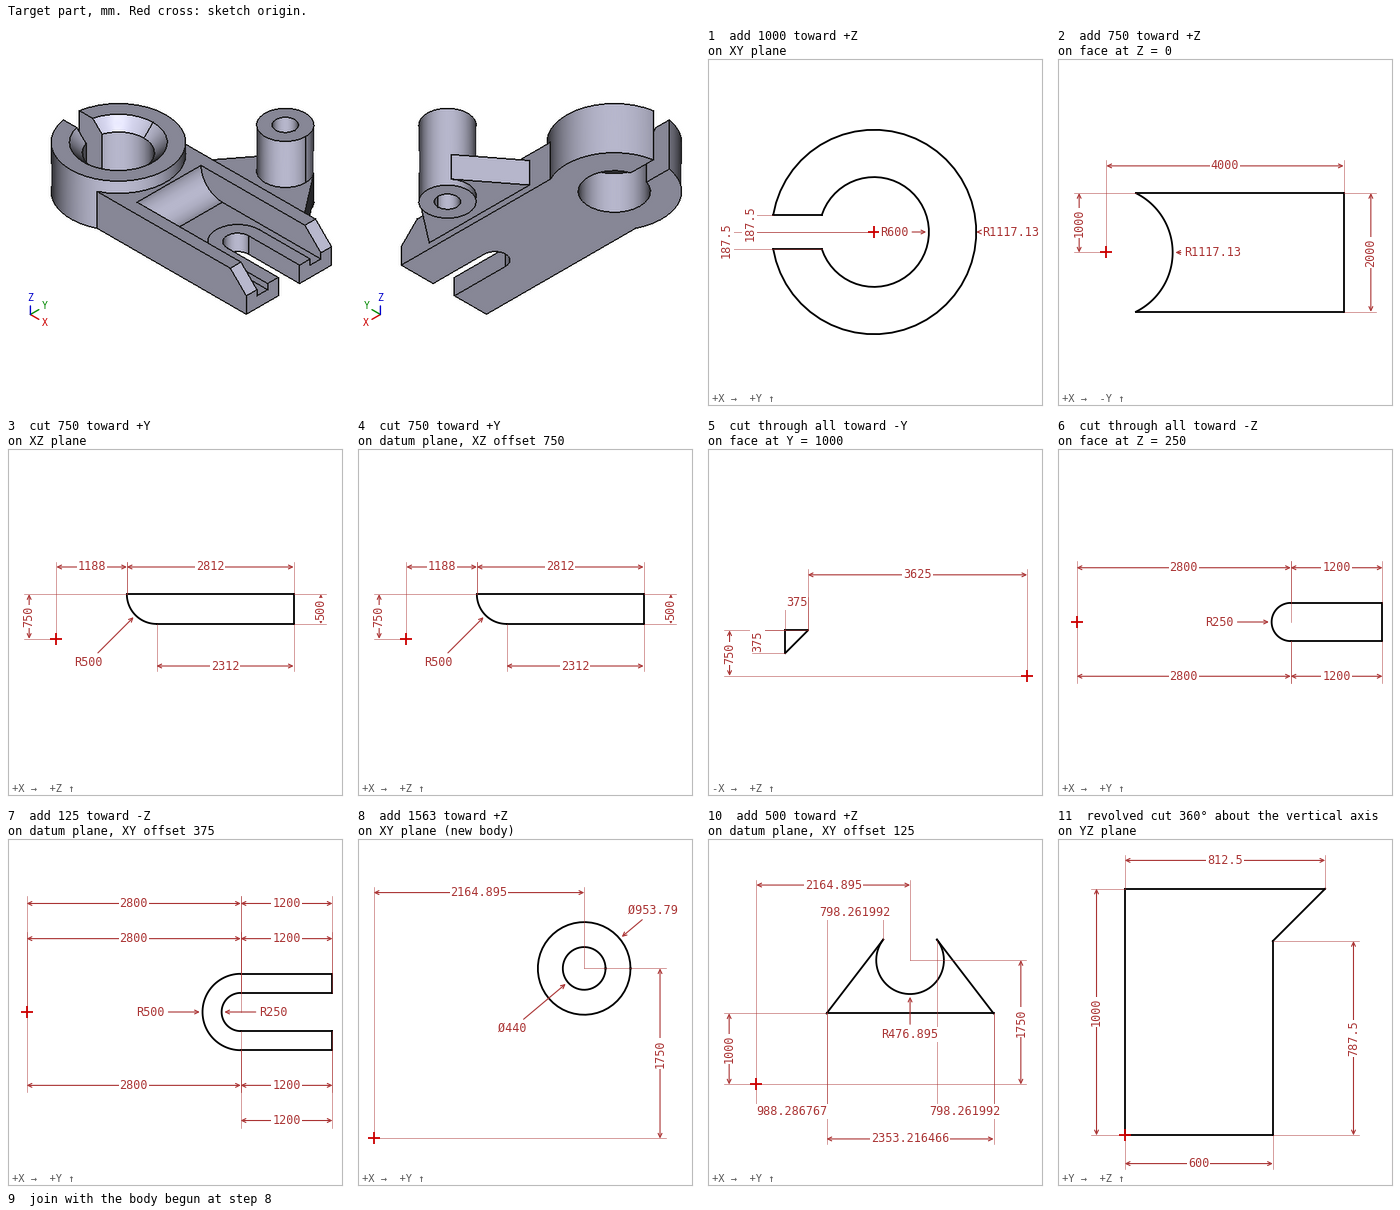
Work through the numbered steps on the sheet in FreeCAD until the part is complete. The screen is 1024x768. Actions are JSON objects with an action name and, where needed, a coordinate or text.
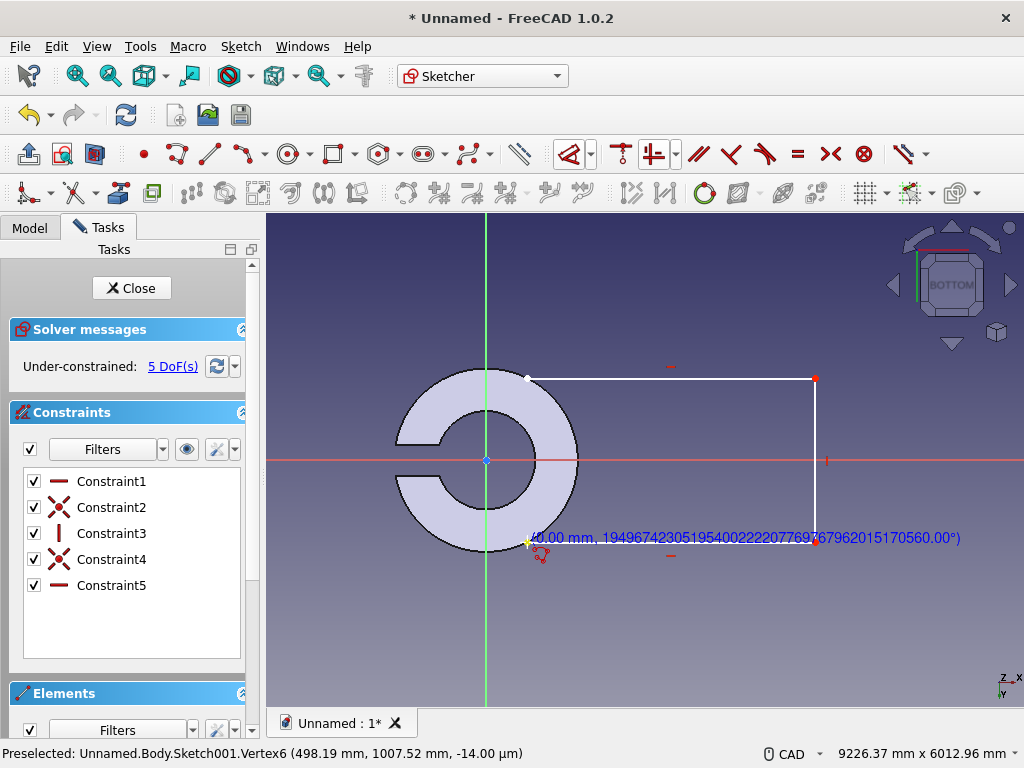
{"action": "key", "text": "g 3 a"}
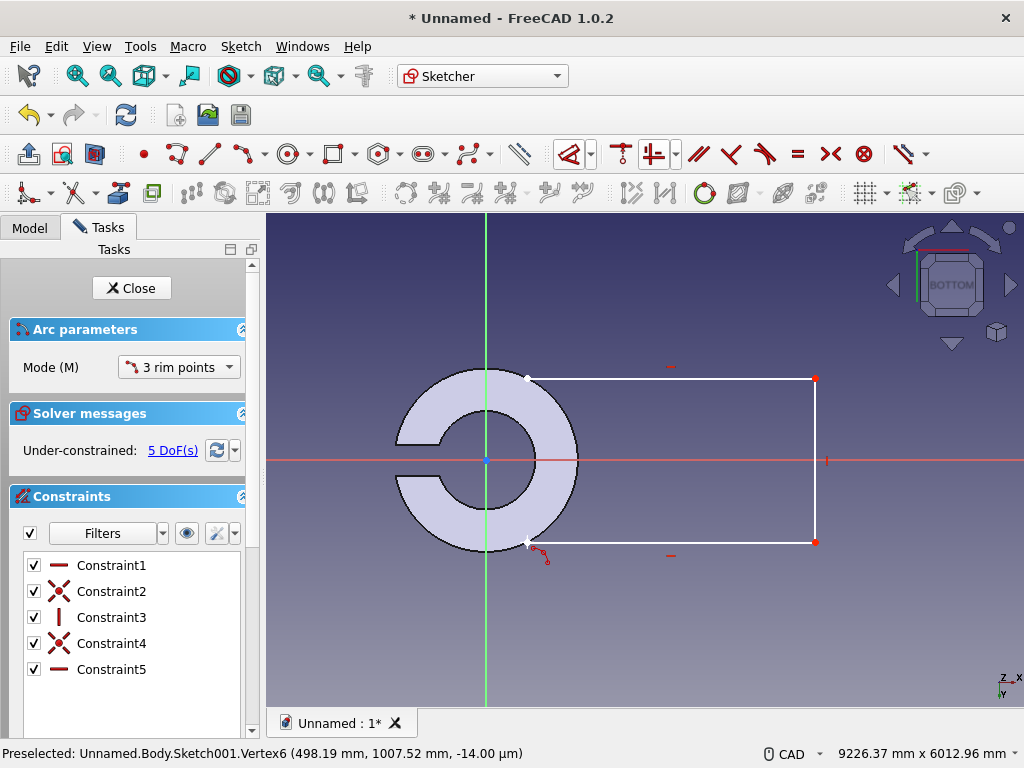
{"action": "left_click", "coordinate": [527, 543]}
{"action": "left_click", "coordinate": [527, 379]}
{"action": "left_click", "coordinate": [576, 480]}
{"action": "key", "text": "Escape"}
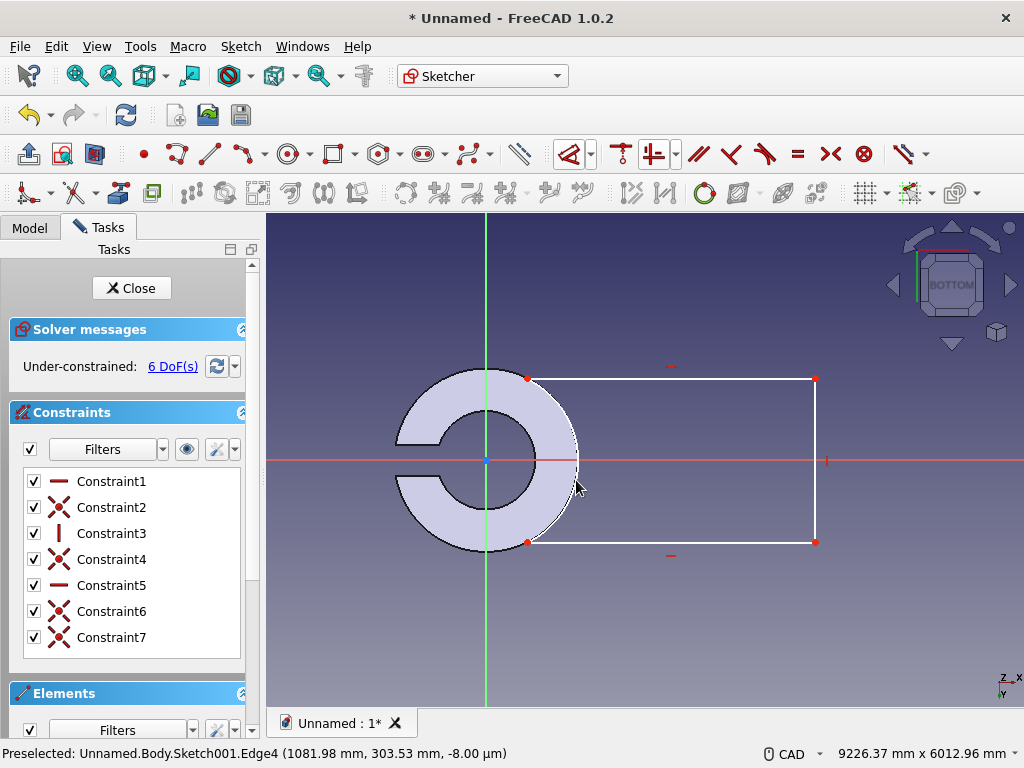
{"action": "left_click_drag", "start_coordinate": [476, 450], "coordinate": [497, 471]}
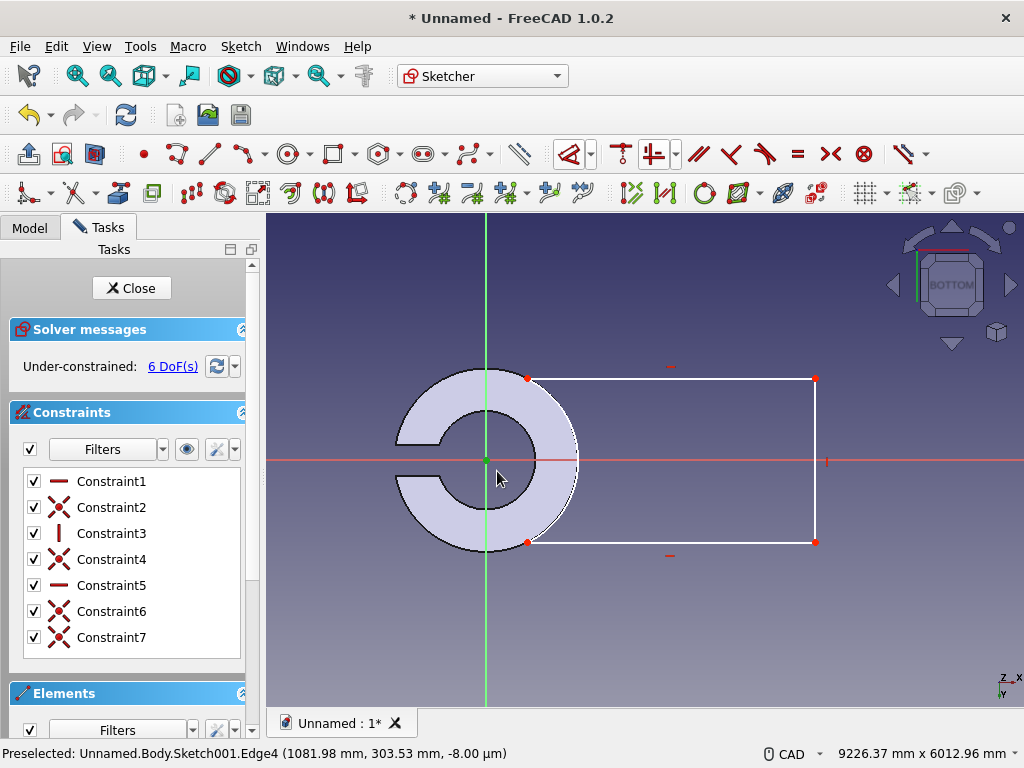
{"action": "left_click", "coordinate": [621, 154]}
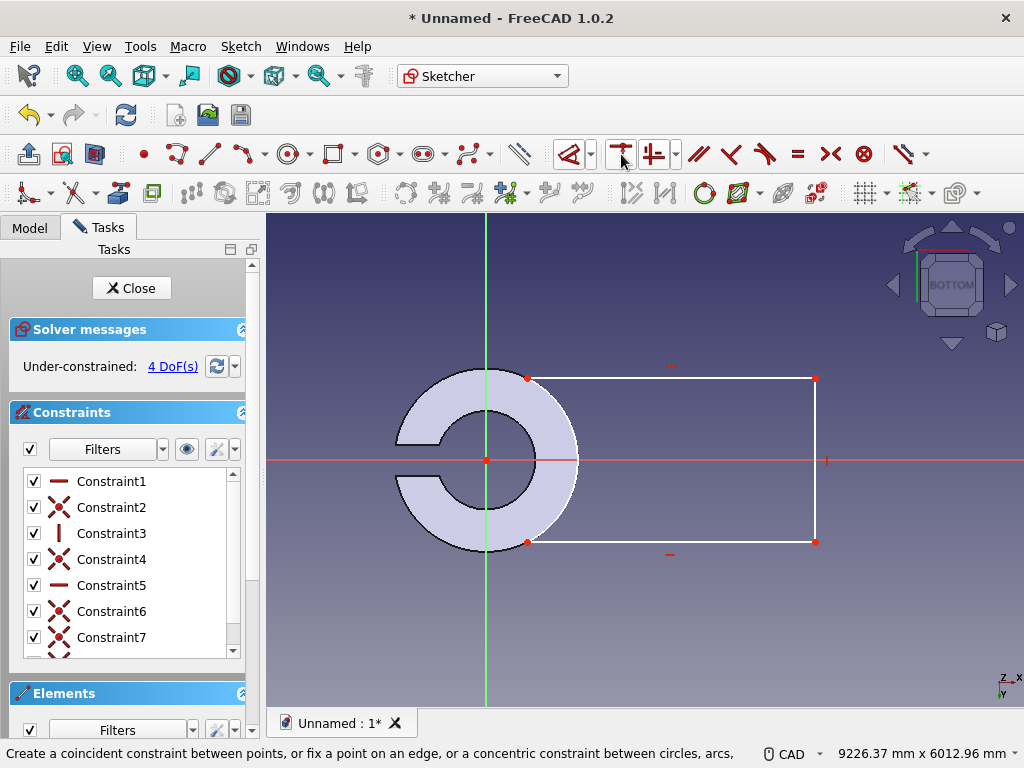
{"action": "left_click", "coordinate": [568, 154]}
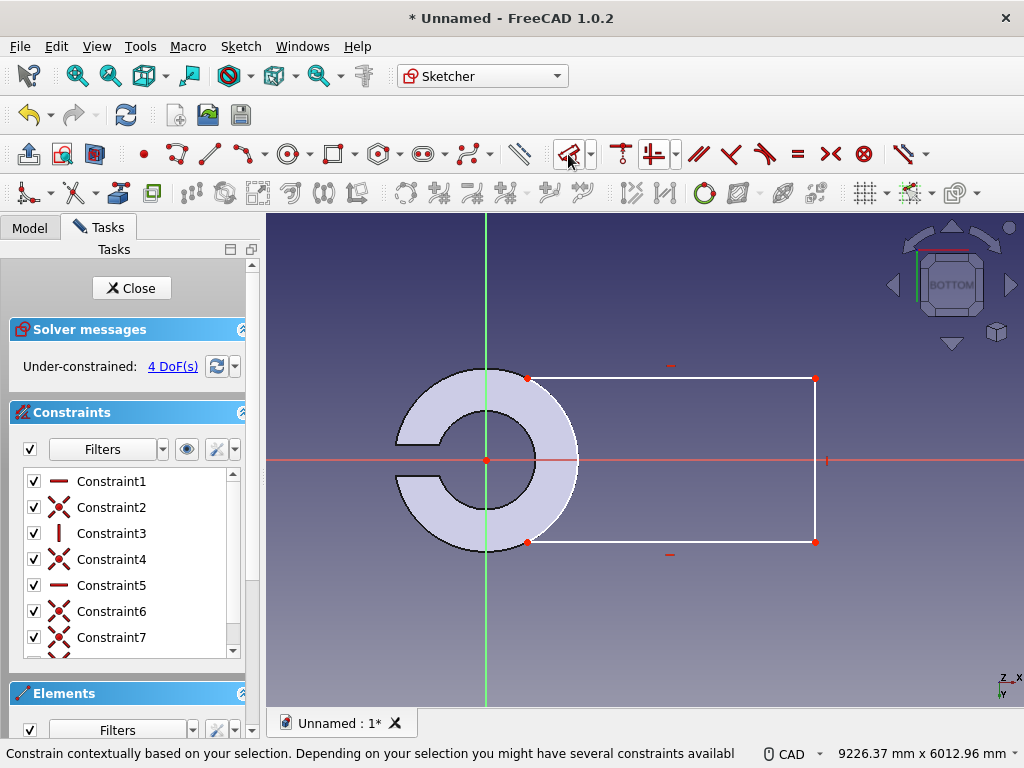
{"action": "left_click", "coordinate": [569, 500]}
{"action": "left_click", "coordinate": [598, 514]}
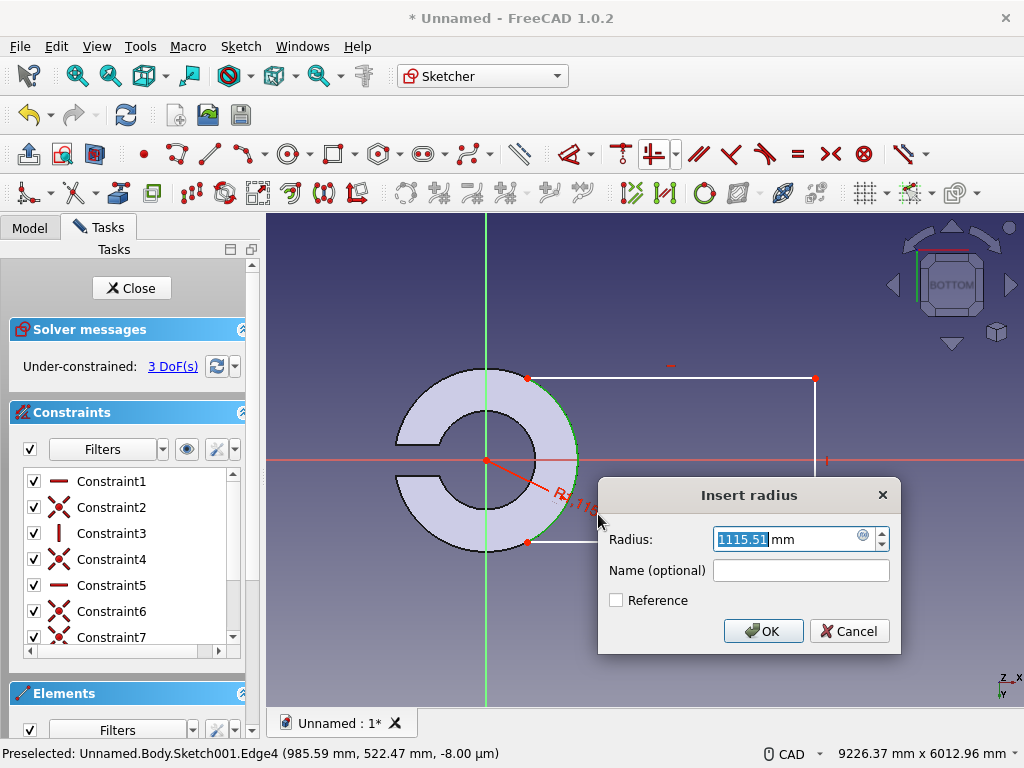
{"action": "type", "text": "1117.13"}
{"action": "key", "text": "Return"}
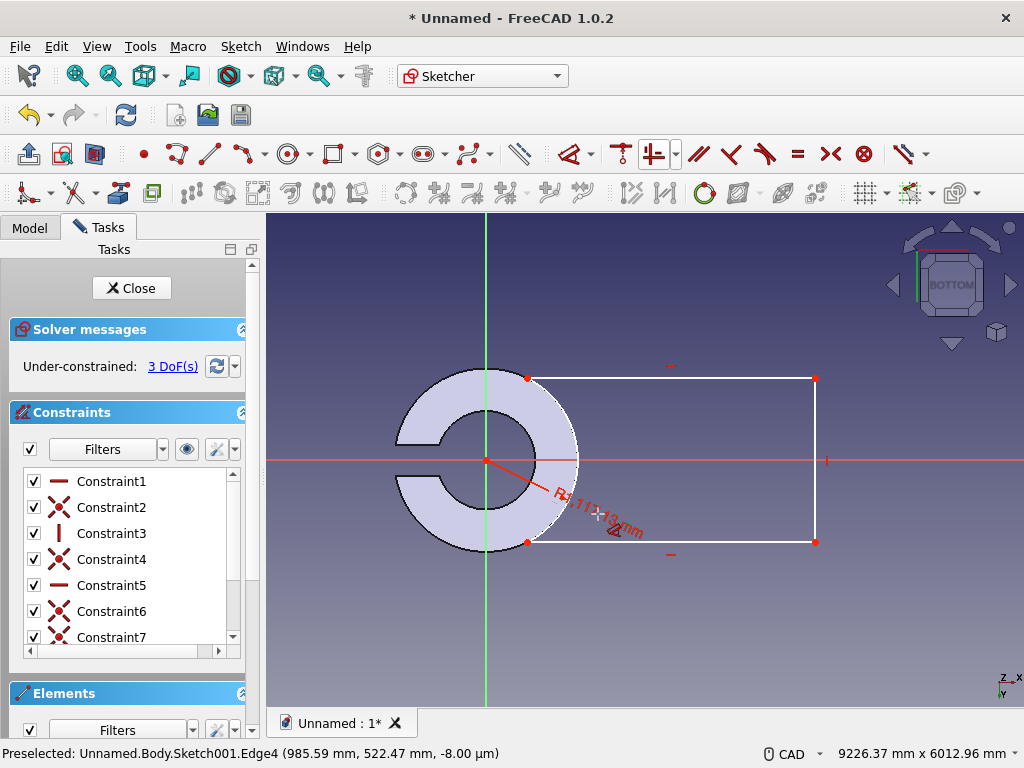
{"action": "left_click", "coordinate": [815, 427]}
{"action": "left_click", "coordinate": [849, 422]}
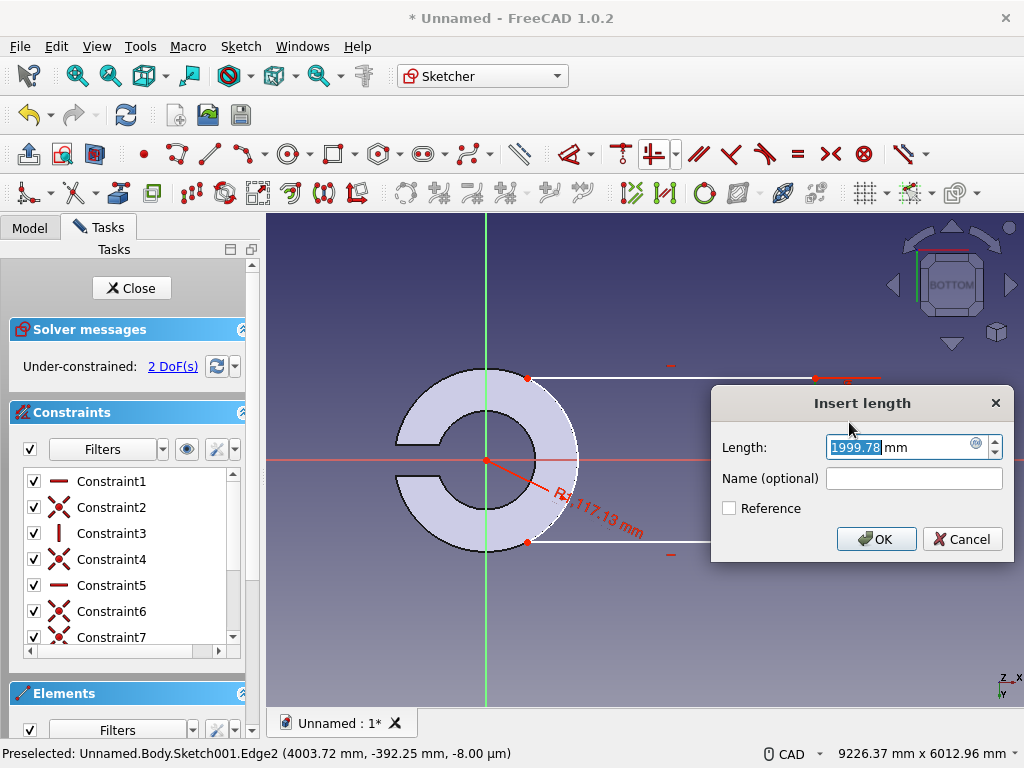
{"action": "type", "text": "2000"}
{"action": "key", "text": "Return"}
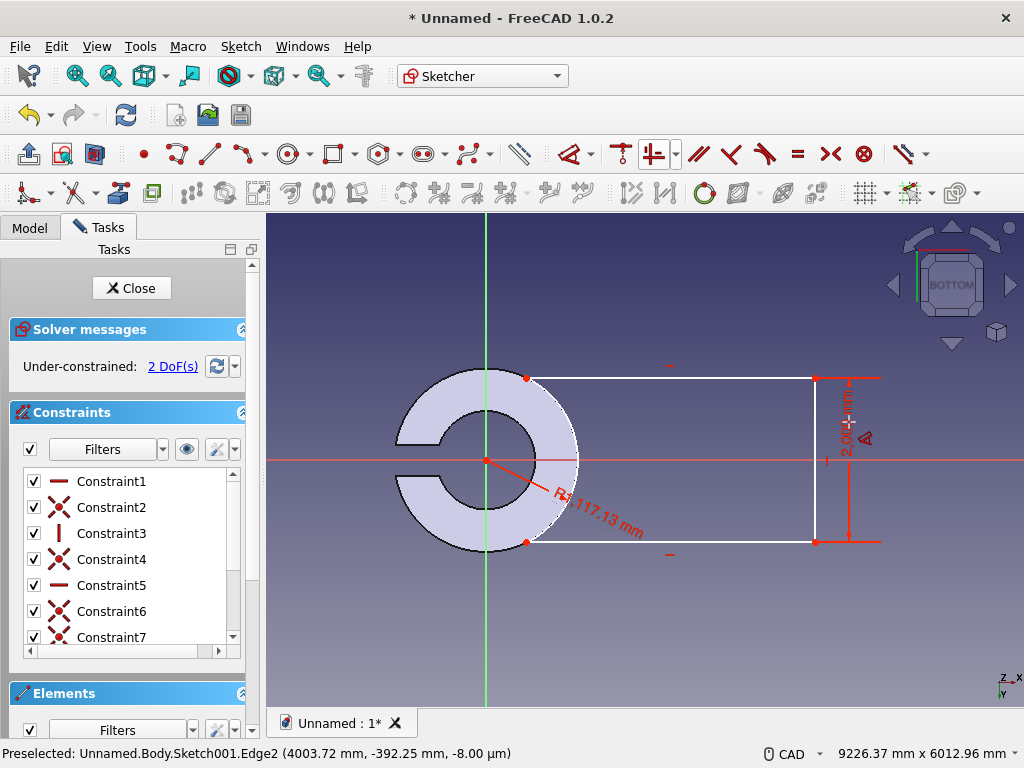
{"action": "left_click", "coordinate": [527, 378]}
{"action": "left_click", "coordinate": [452, 419]}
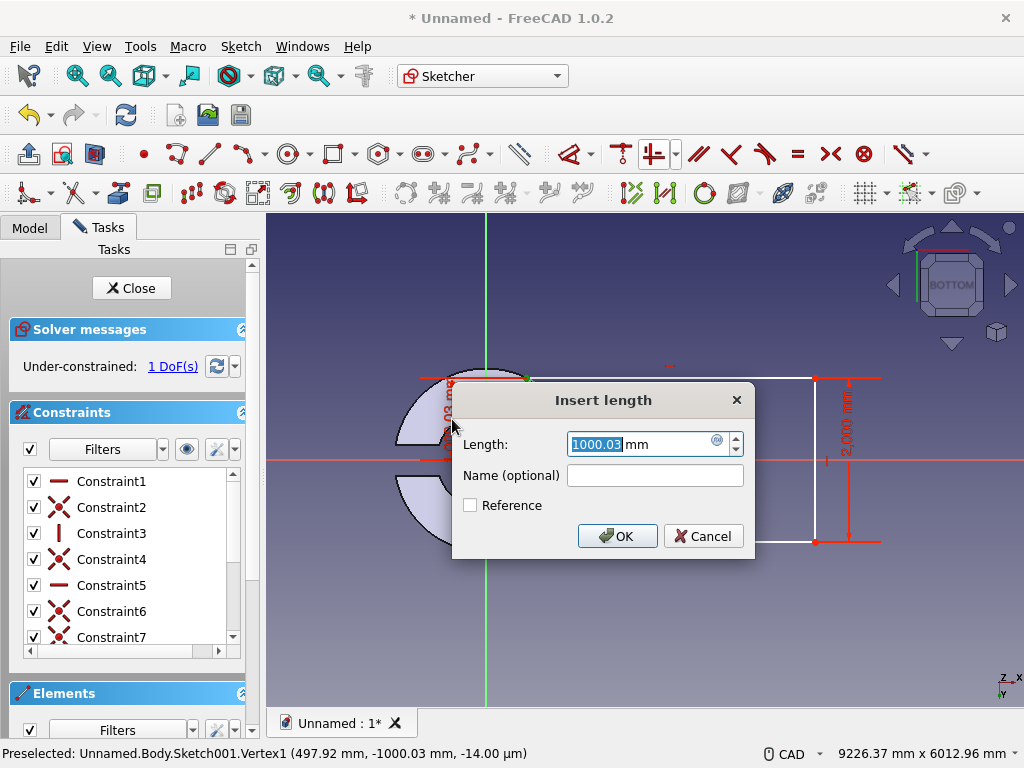
{"action": "type", "text": "1000"}
{"action": "key", "text": "Return"}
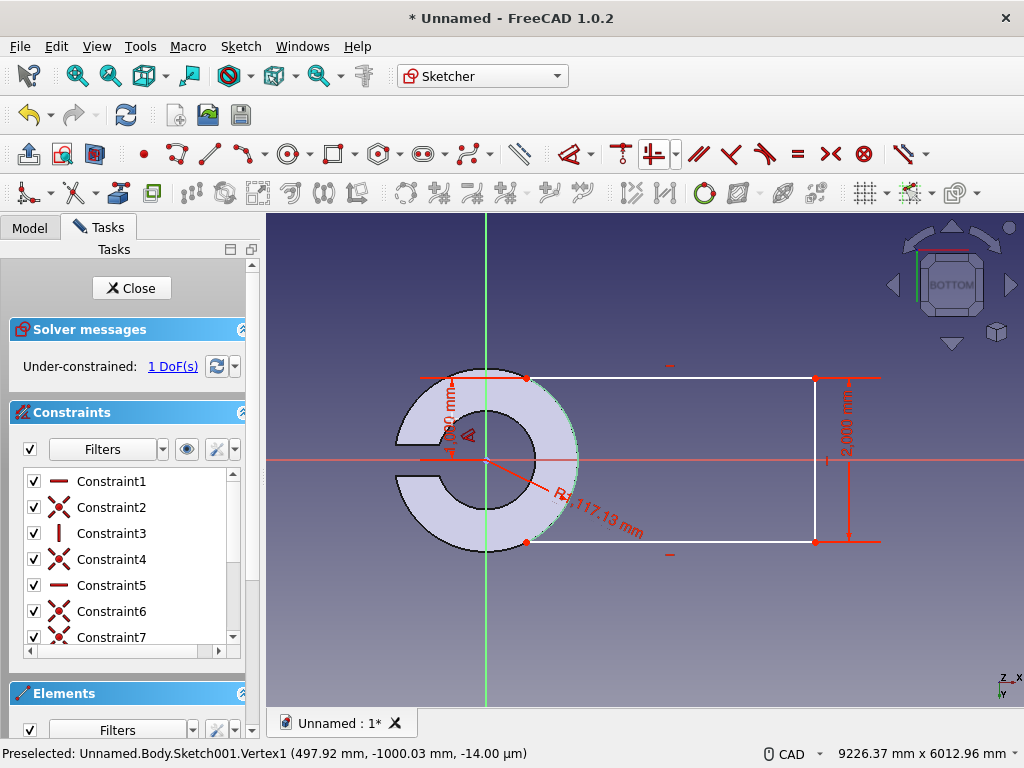
{"action": "left_click", "coordinate": [815, 378]}
{"action": "left_click", "coordinate": [651, 344]}